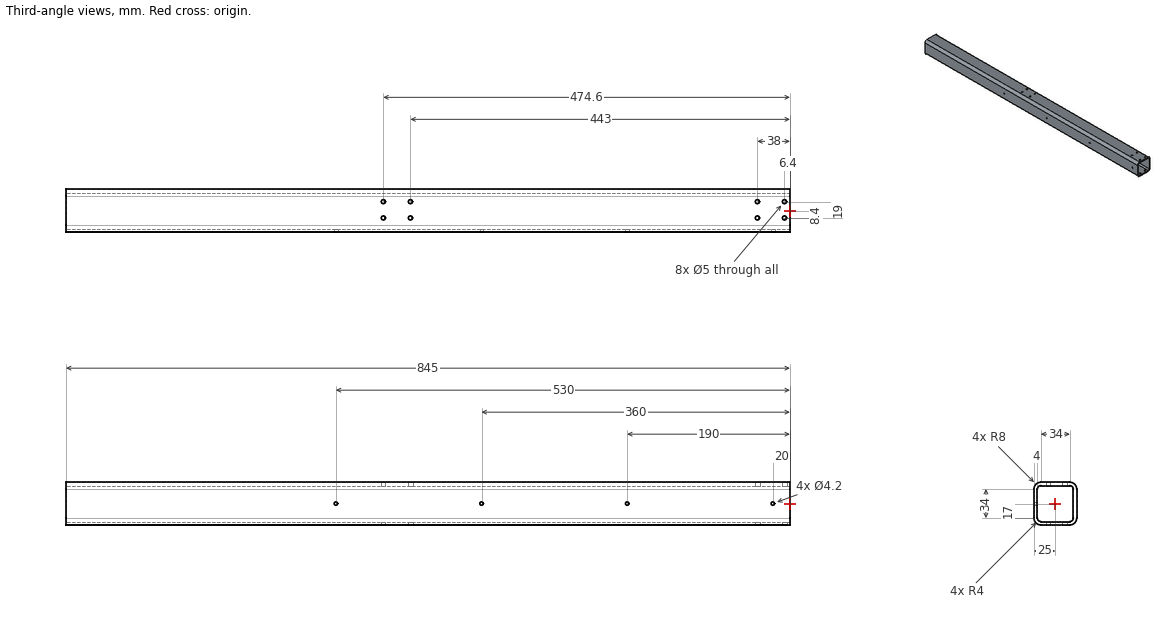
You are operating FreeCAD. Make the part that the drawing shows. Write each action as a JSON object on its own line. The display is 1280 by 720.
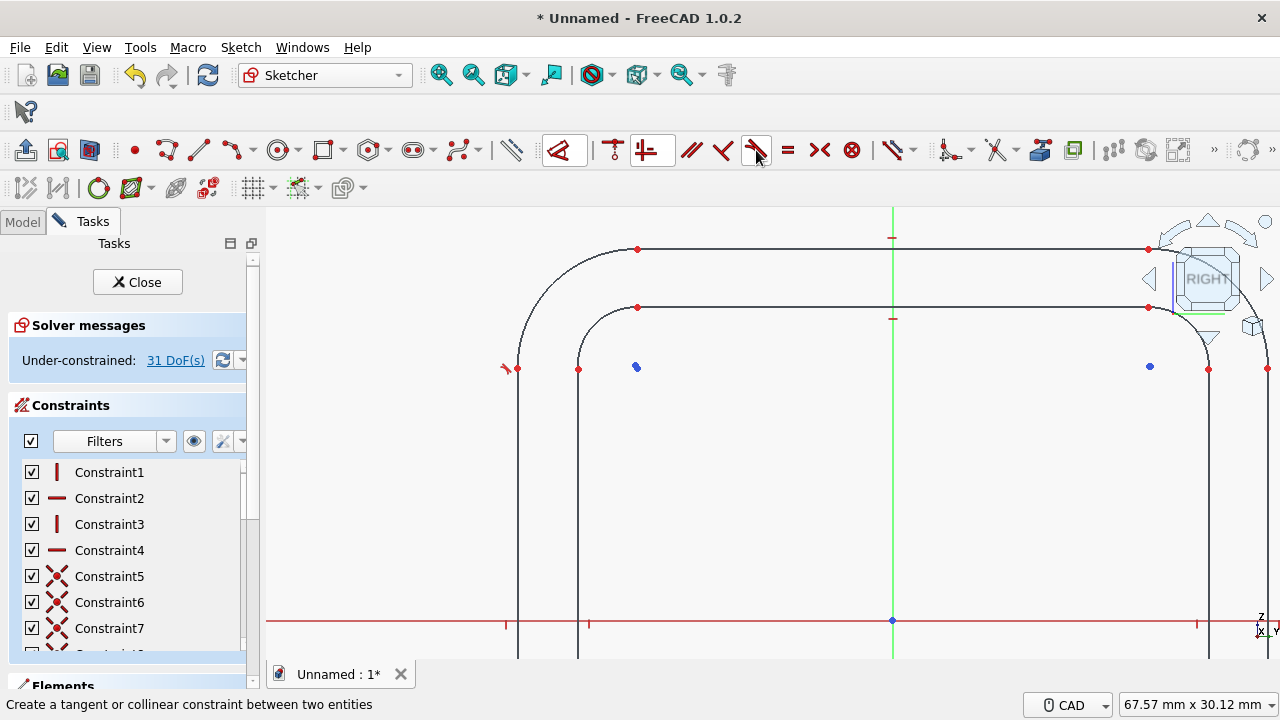
{"action": "left_click", "coordinate": [518, 522]}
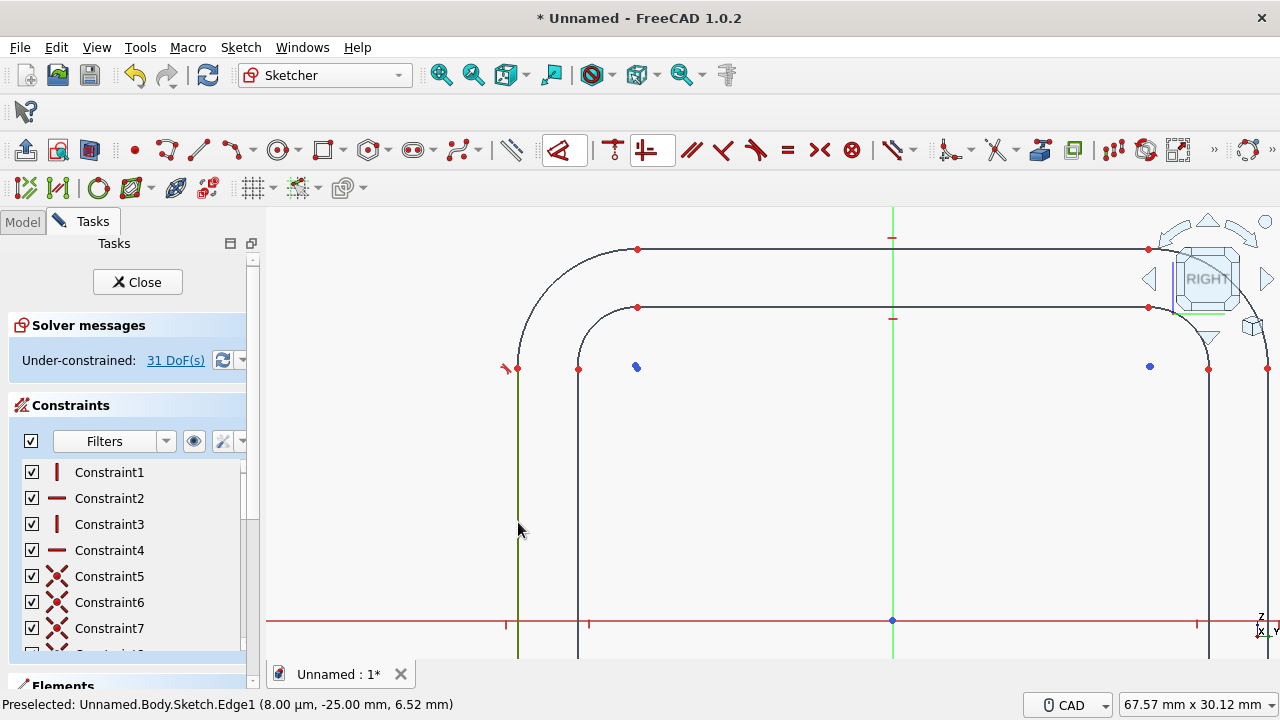
{"action": "scroll", "coordinate": [595, 324], "scroll_direction": "down", "scroll_amount": 5}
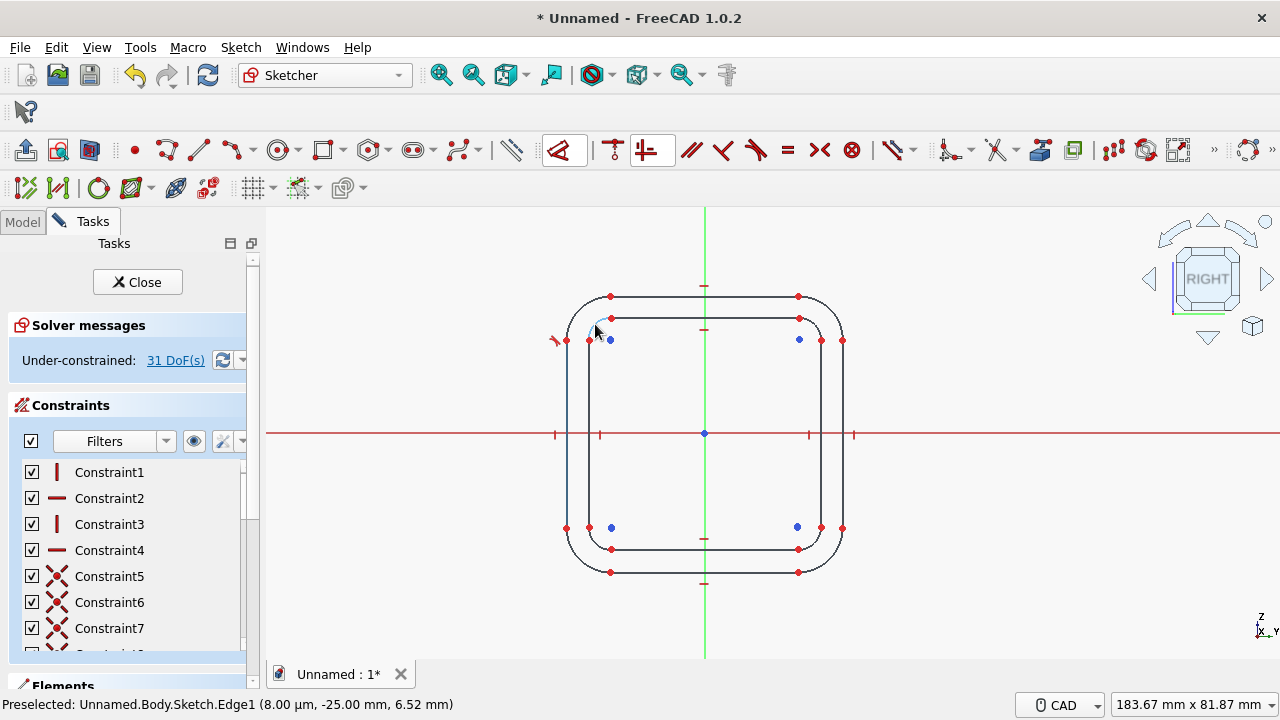
{"action": "left_click", "coordinate": [572, 548]}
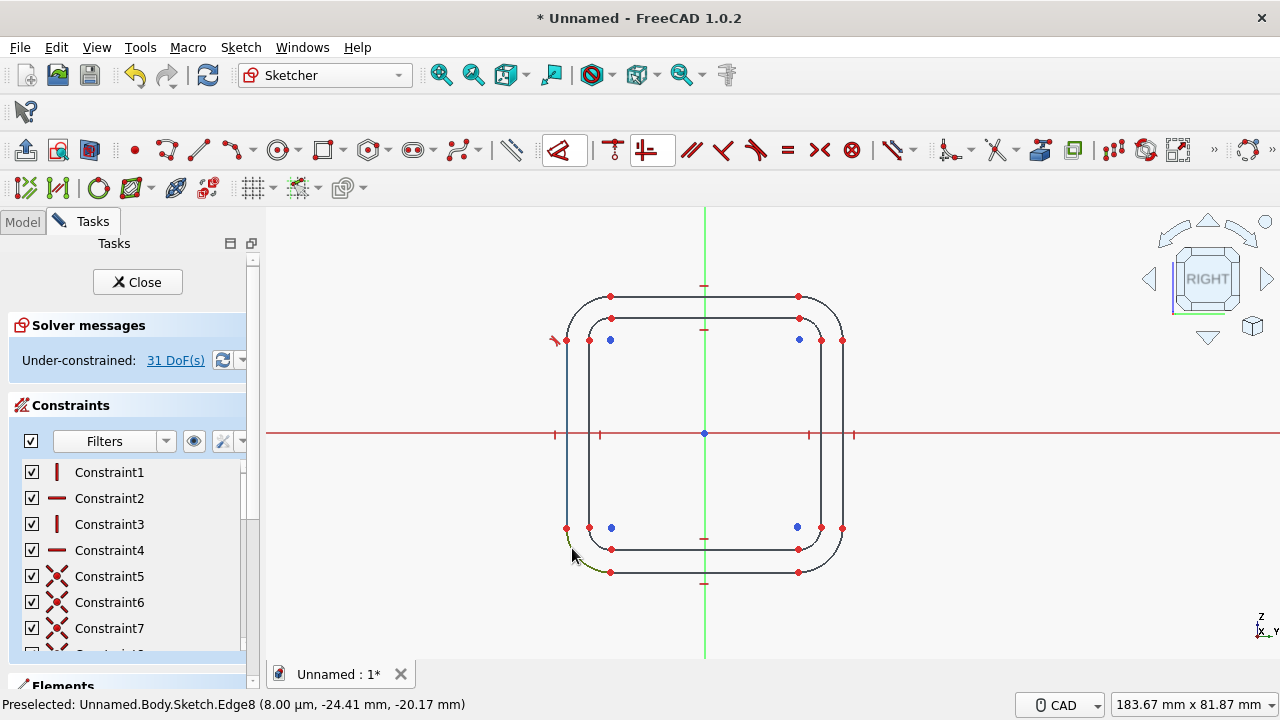
{"action": "left_click", "coordinate": [756, 150]}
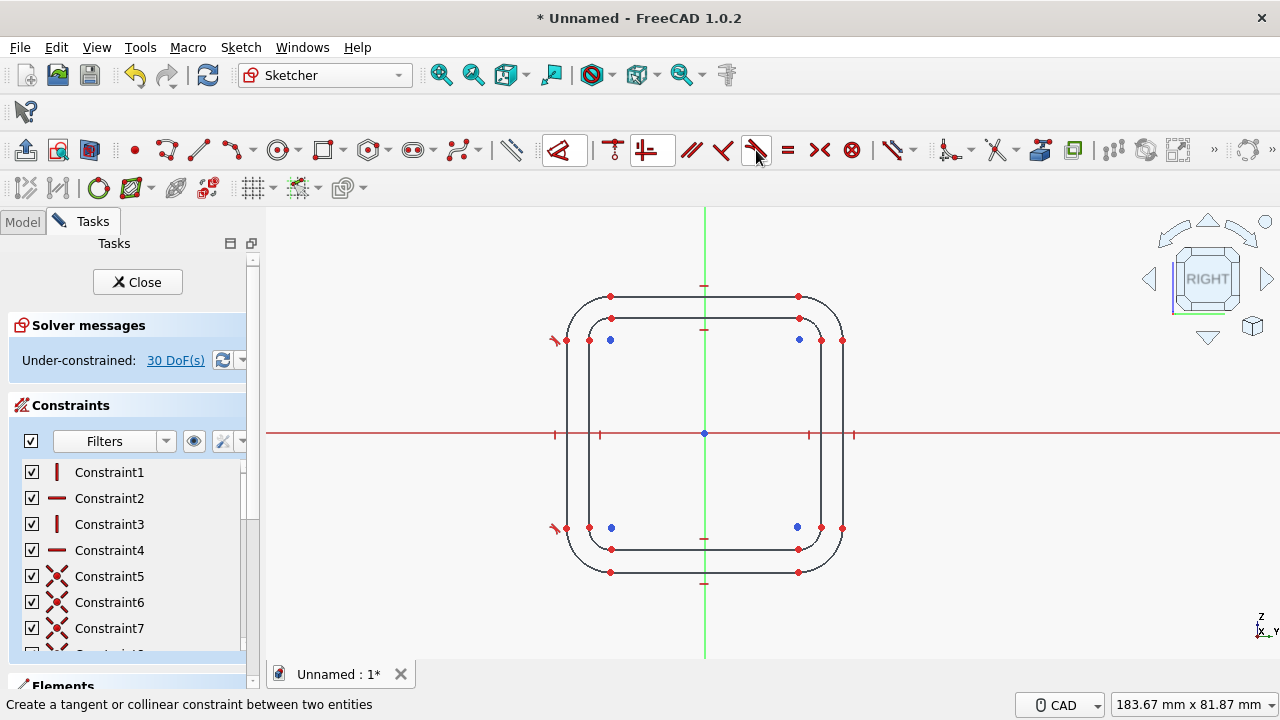
{"action": "left_click", "coordinate": [667, 297]}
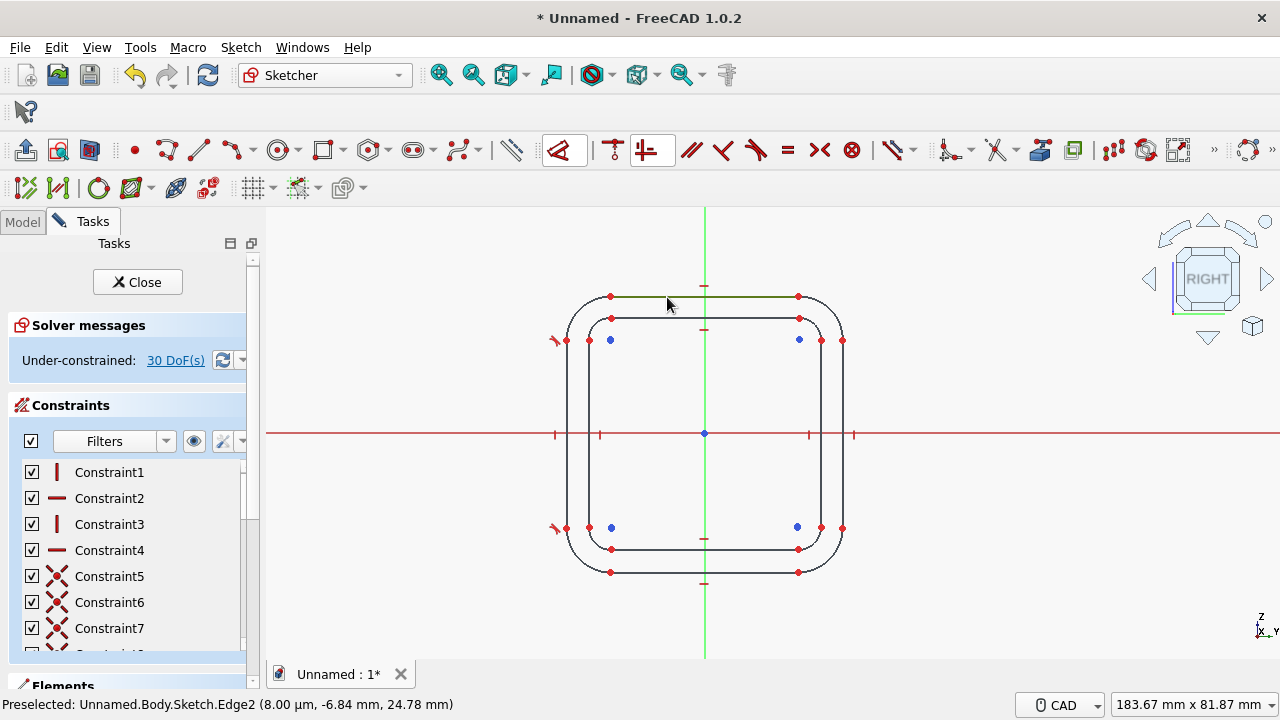
{"action": "left_click", "coordinate": [591, 301]}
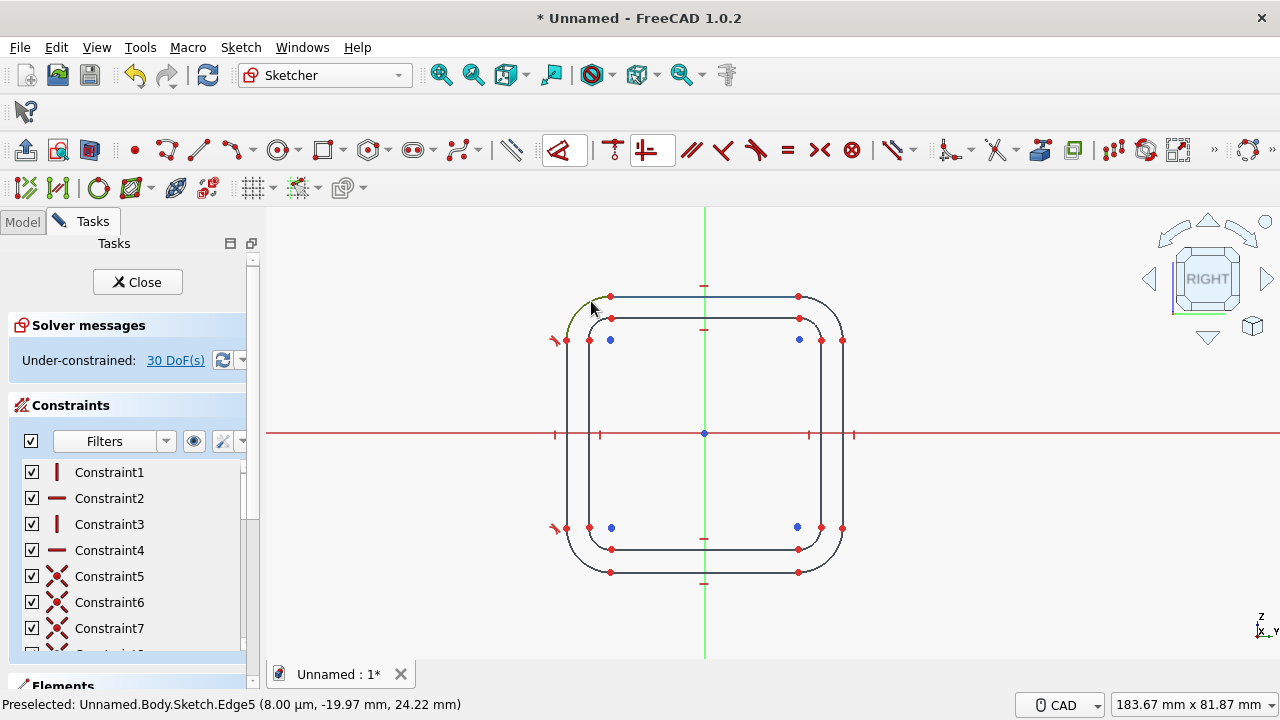
{"action": "left_click", "coordinate": [756, 150]}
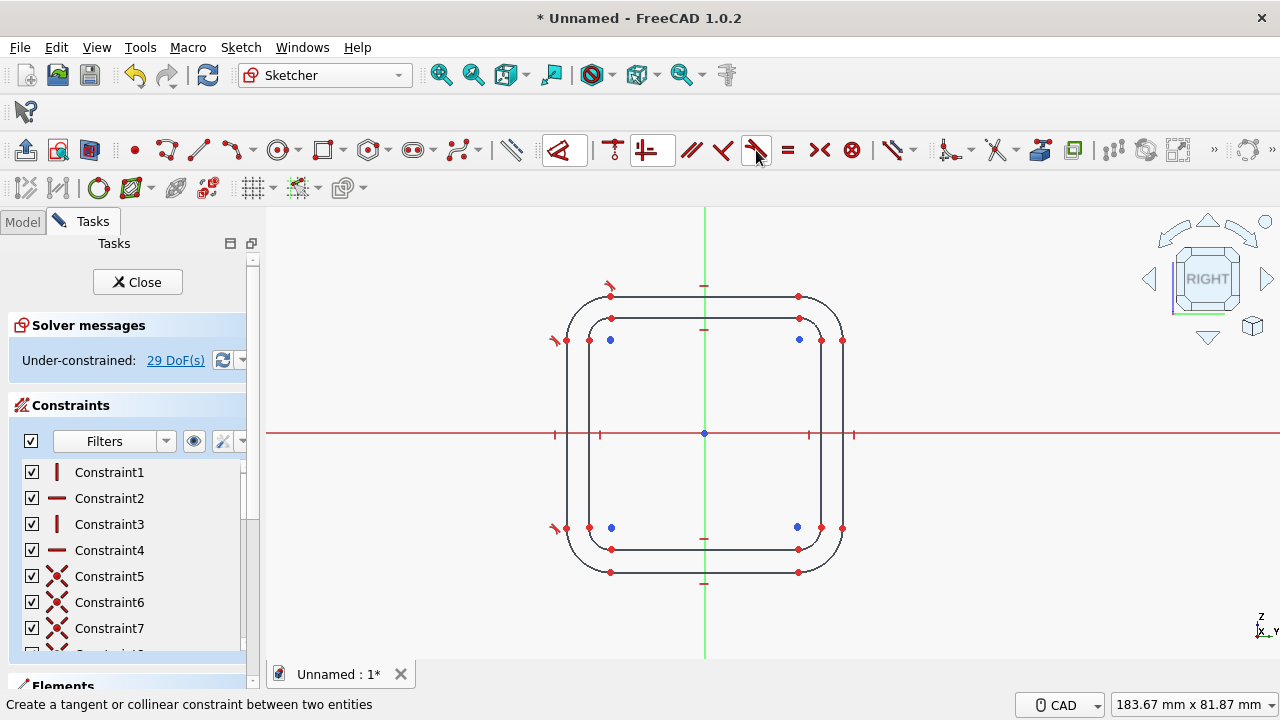
{"action": "left_click", "coordinate": [667, 297]}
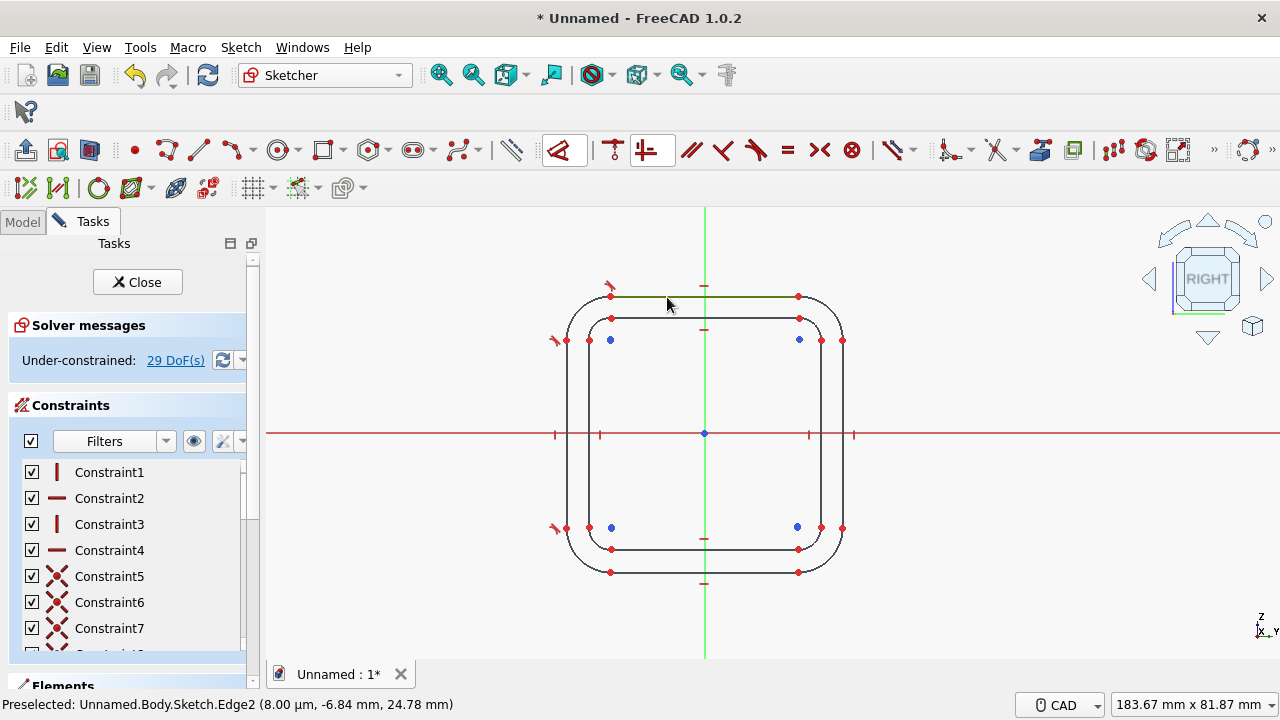
{"action": "left_click", "coordinate": [838, 320]}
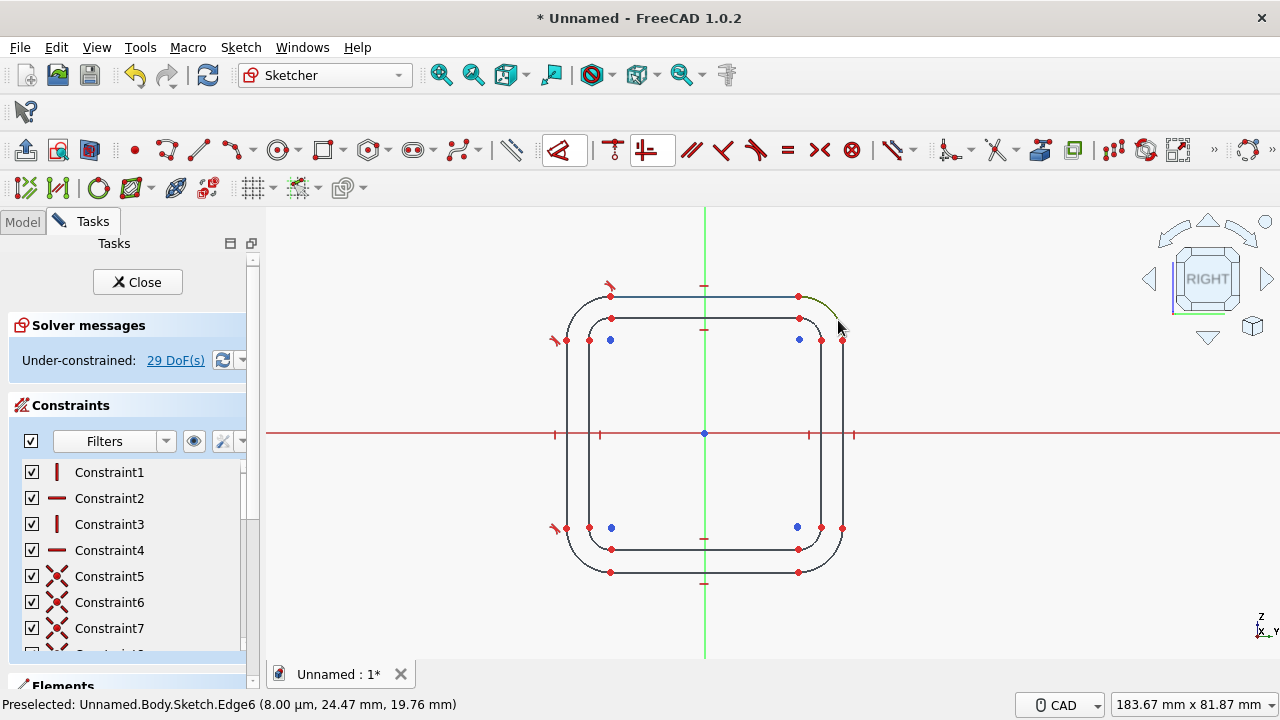
{"action": "left_click", "coordinate": [756, 150]}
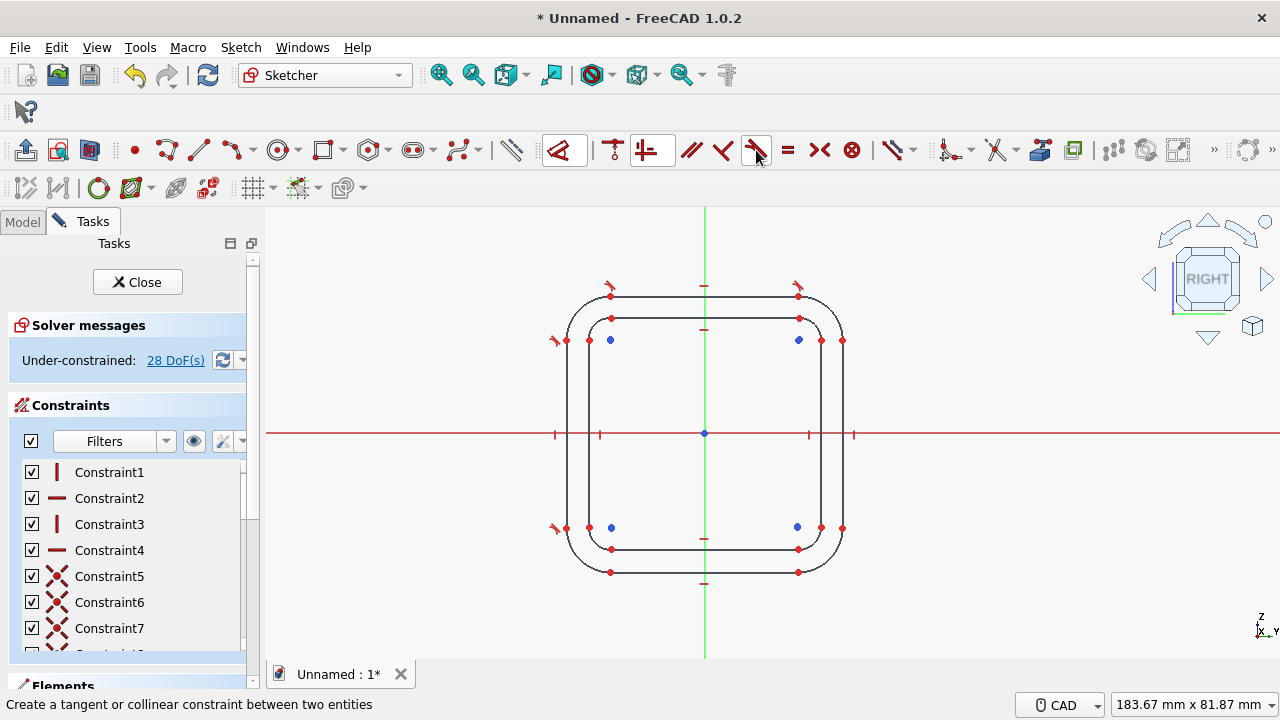
{"action": "left_click", "coordinate": [843, 397]}